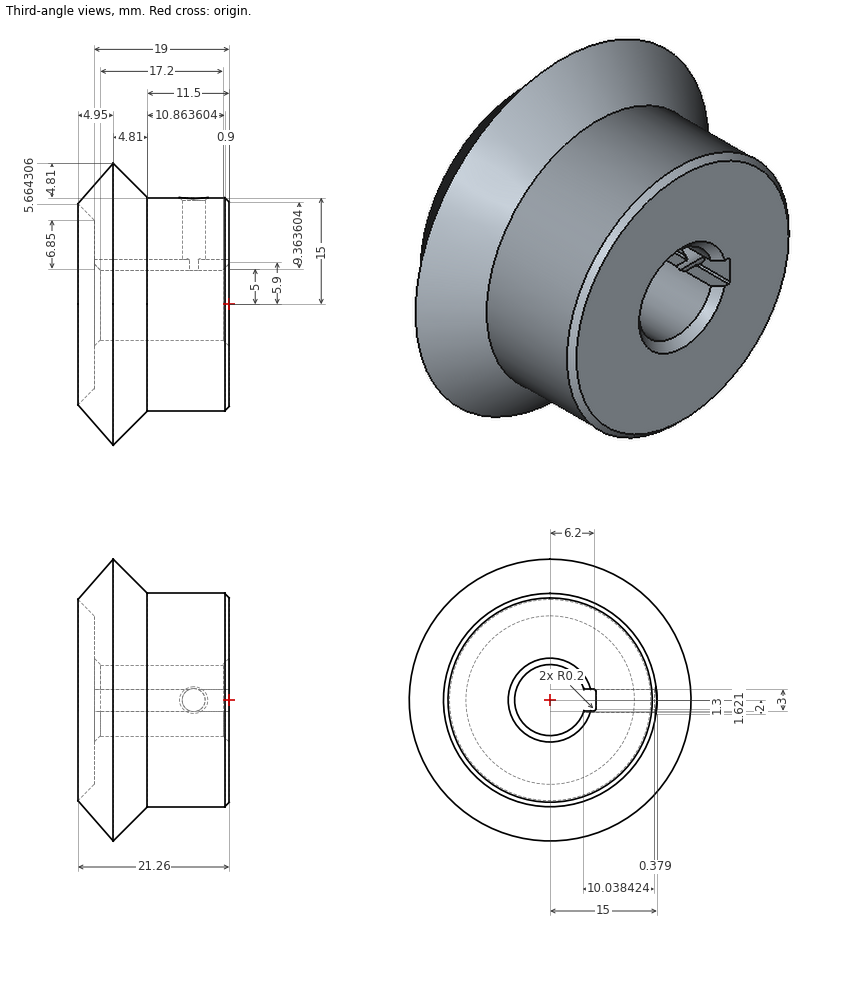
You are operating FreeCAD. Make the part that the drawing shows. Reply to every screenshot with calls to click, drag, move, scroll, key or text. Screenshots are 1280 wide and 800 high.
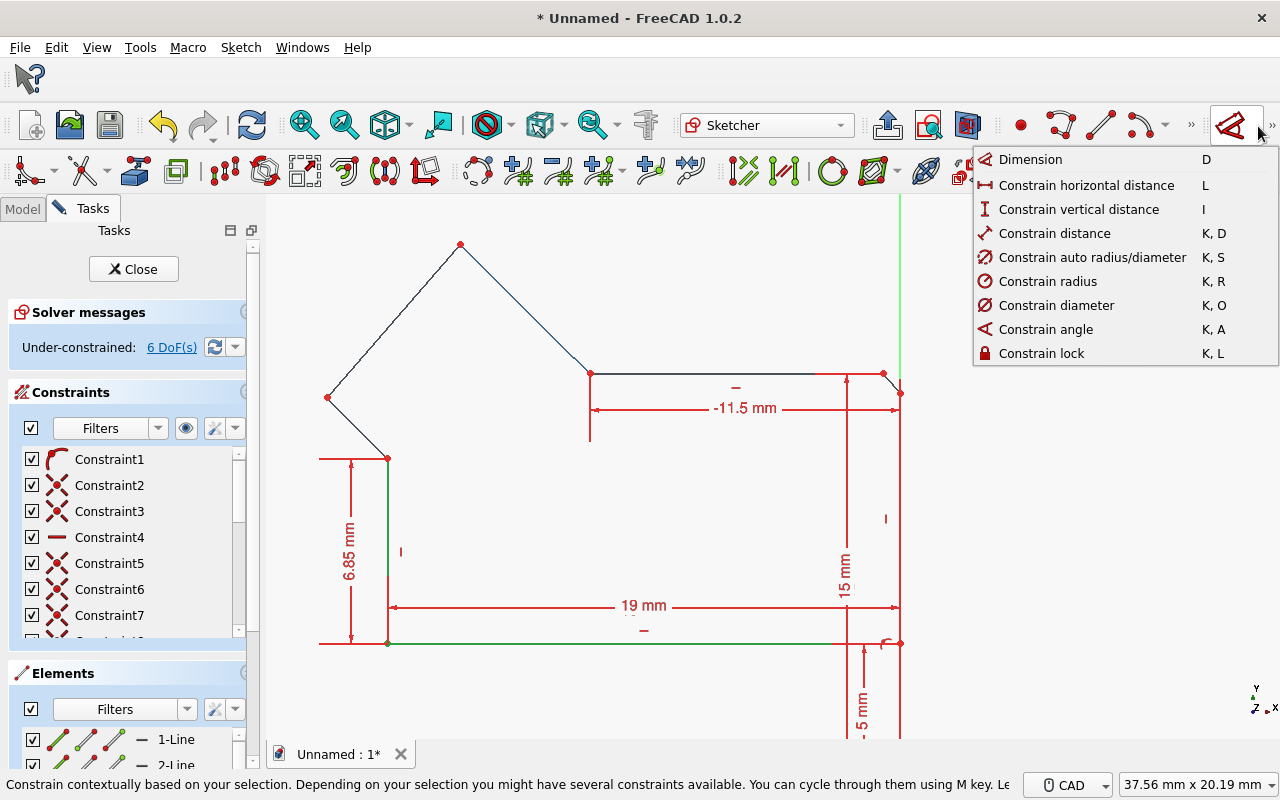
click(1126, 185)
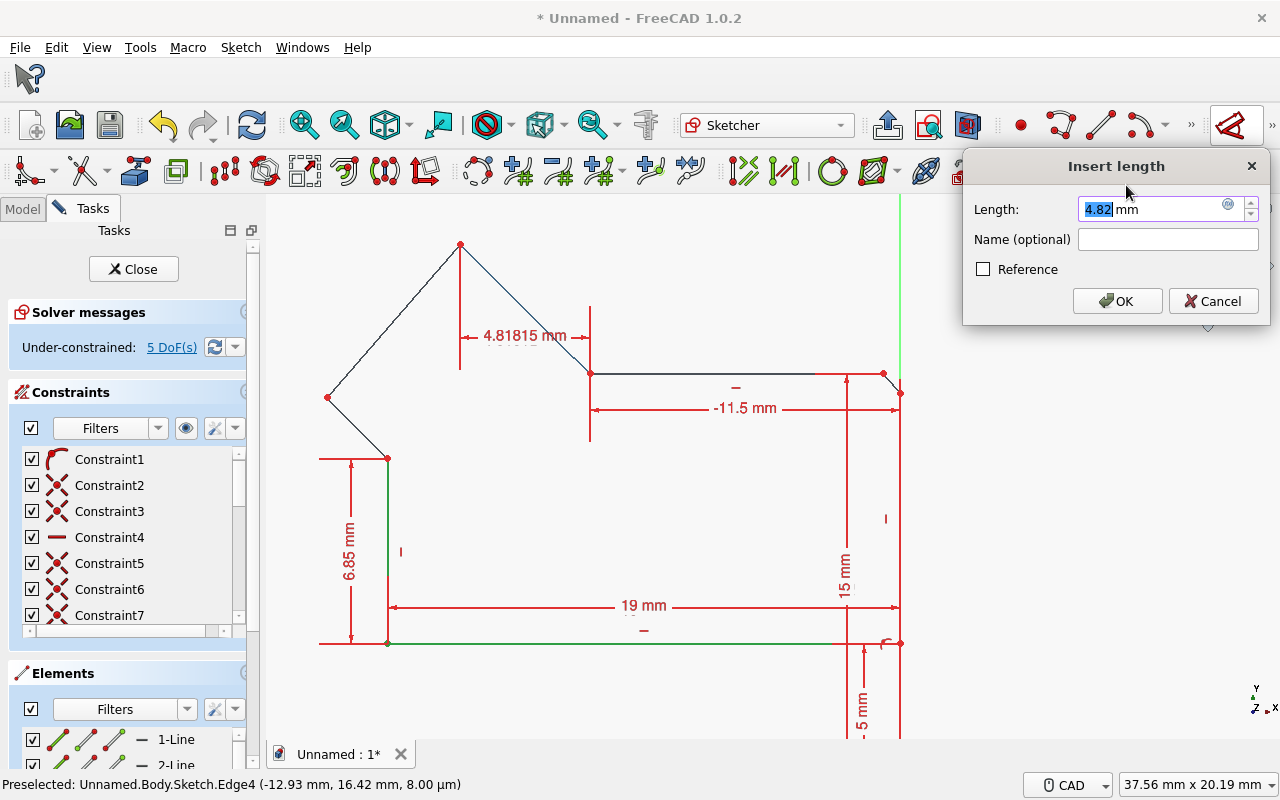
text(4.81)
key(Return)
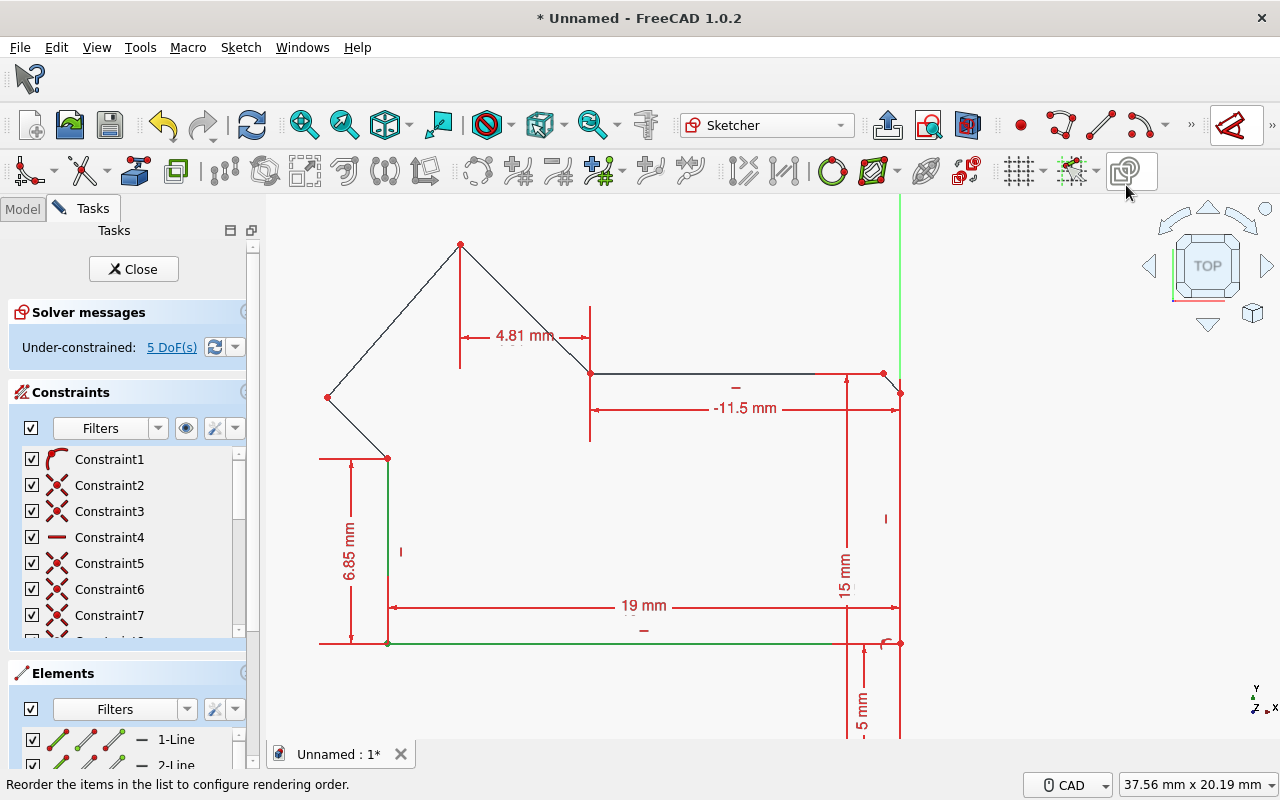
click(499, 284)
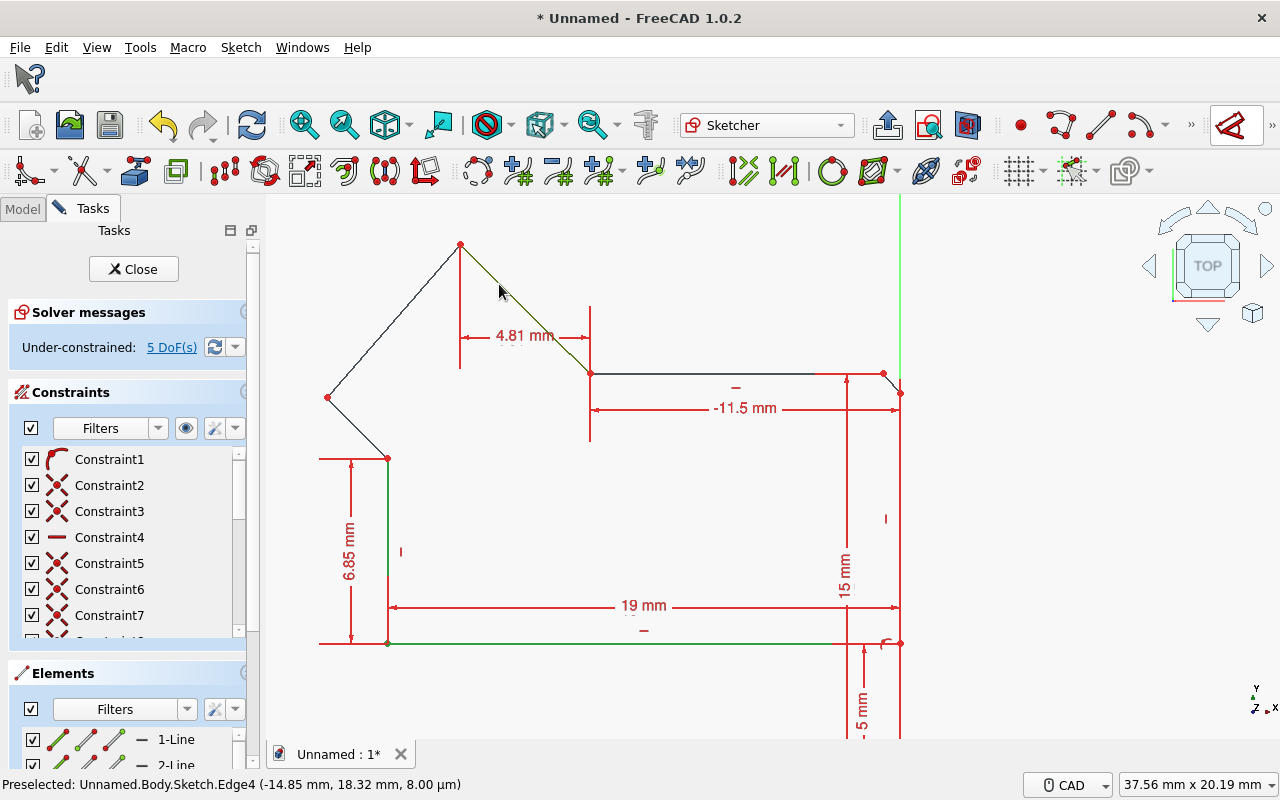
key(i)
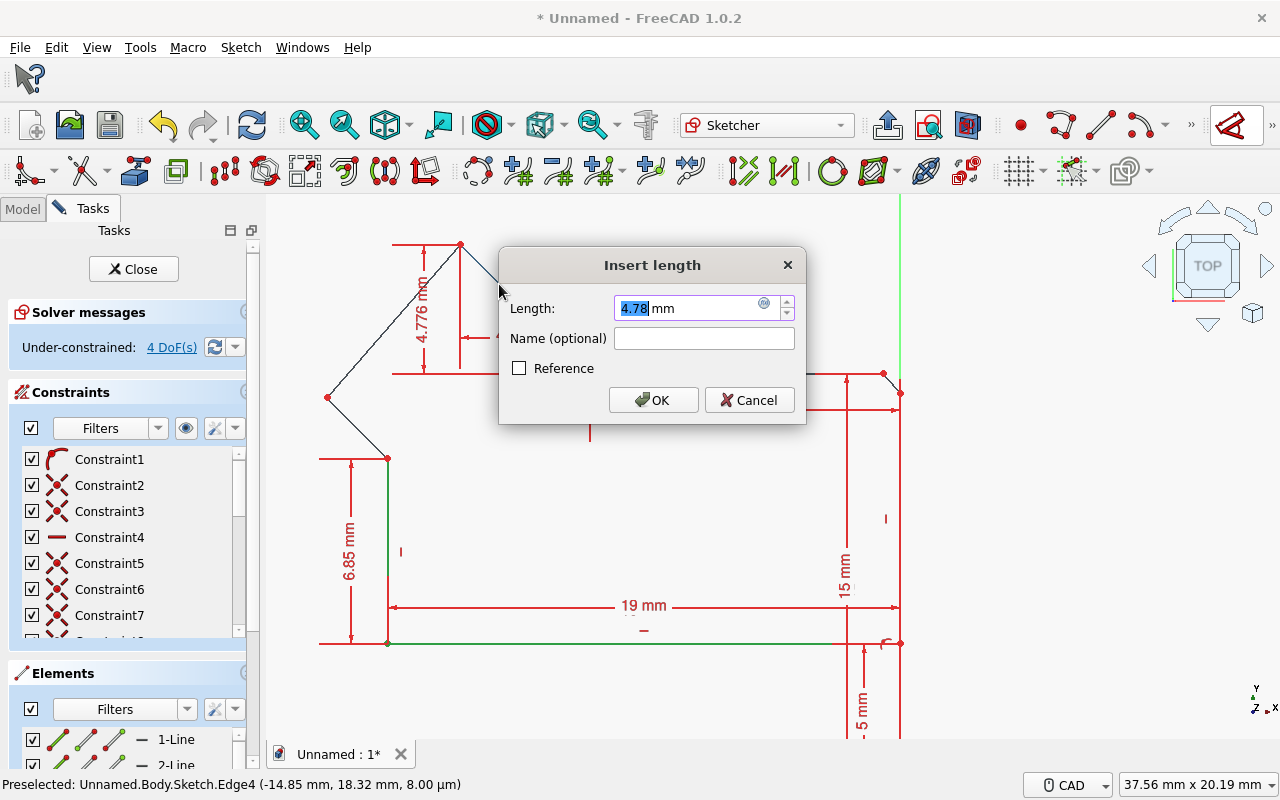
text(4.81)
key(Return)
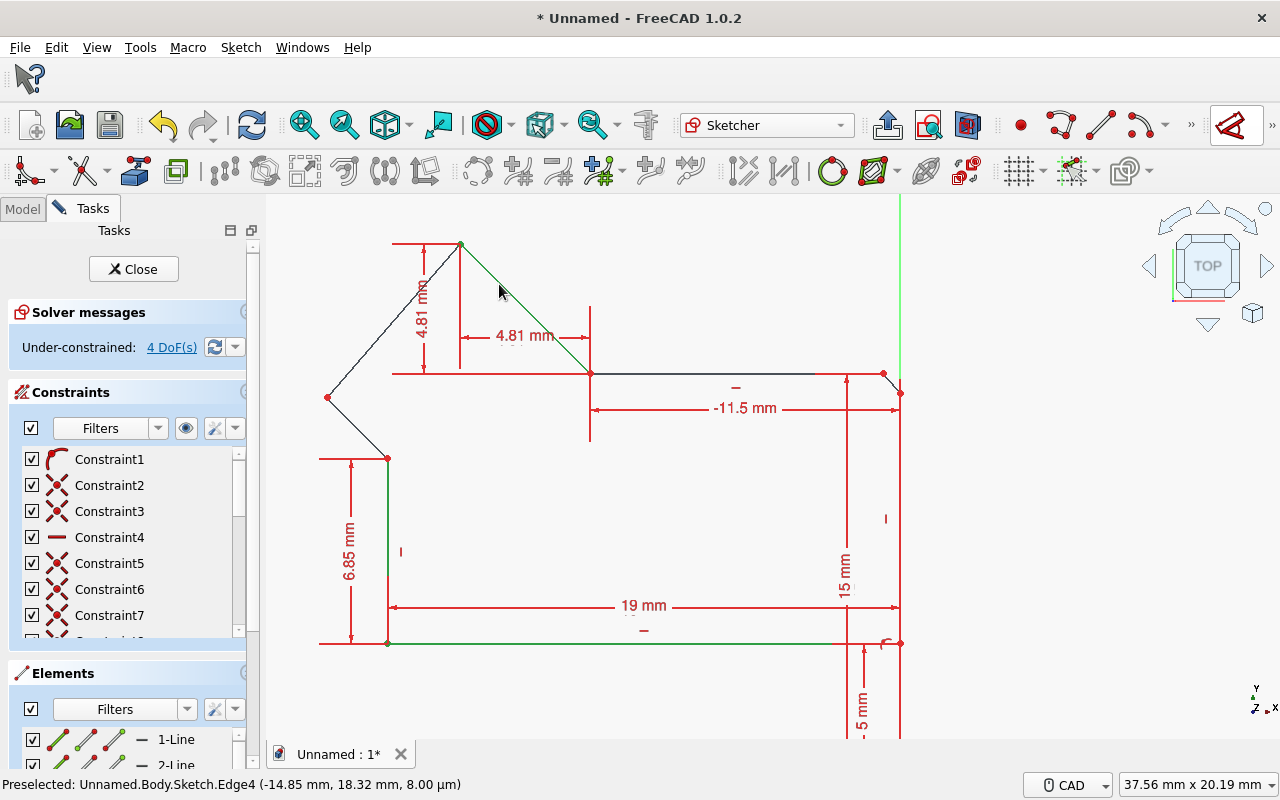
click(367, 352)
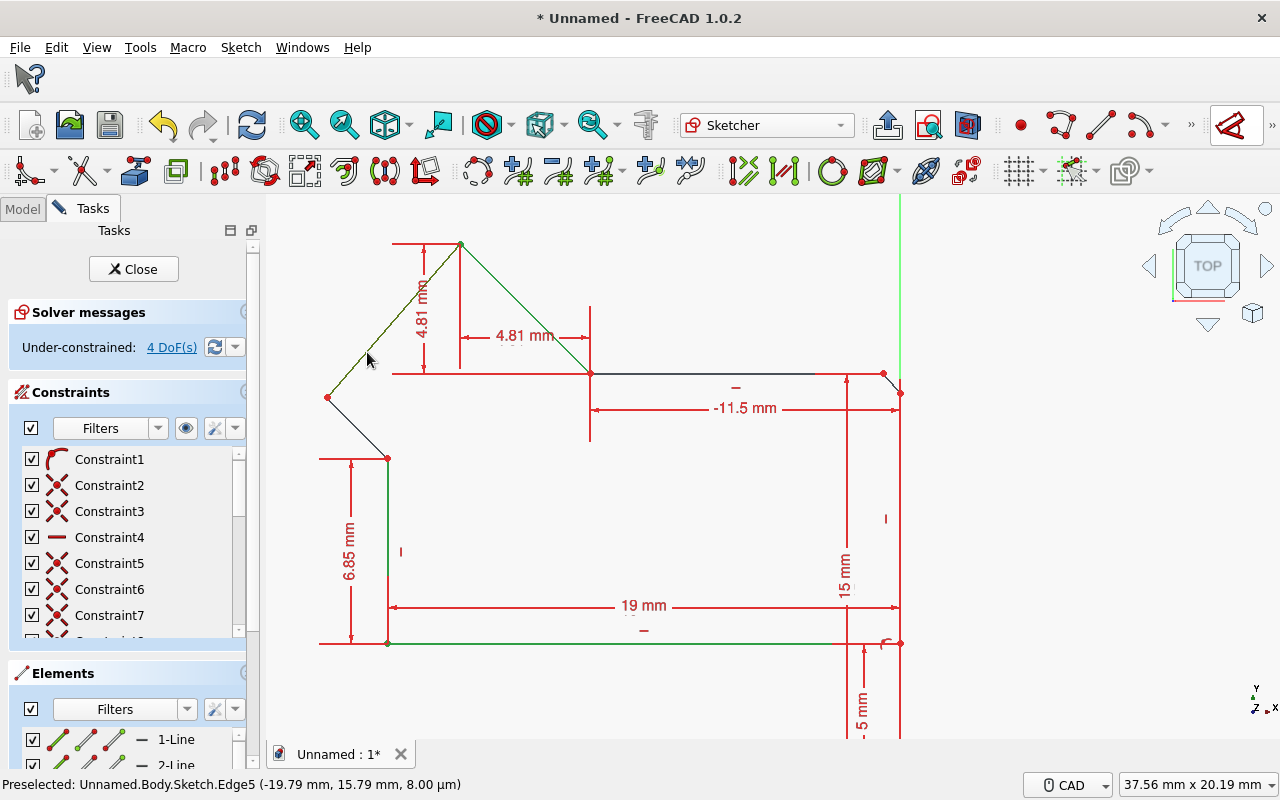
click(1258, 126)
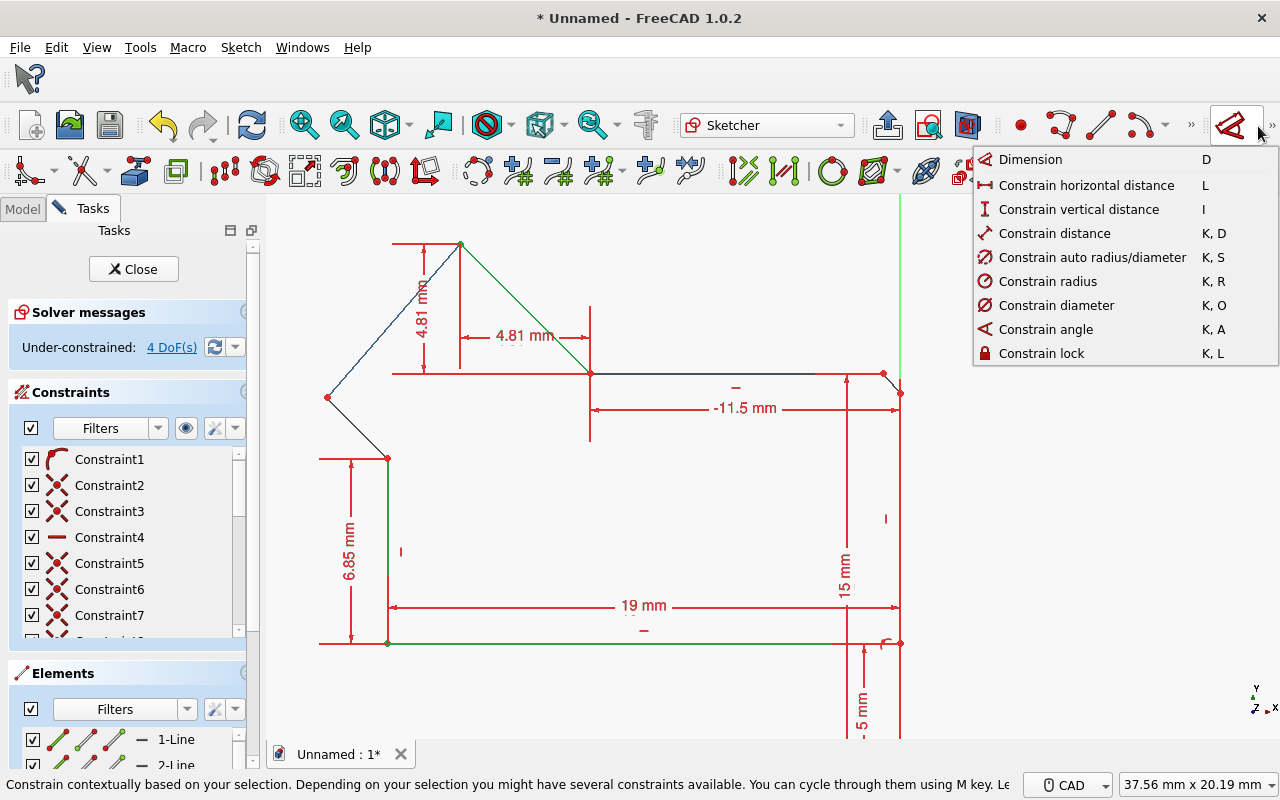
click(1126, 185)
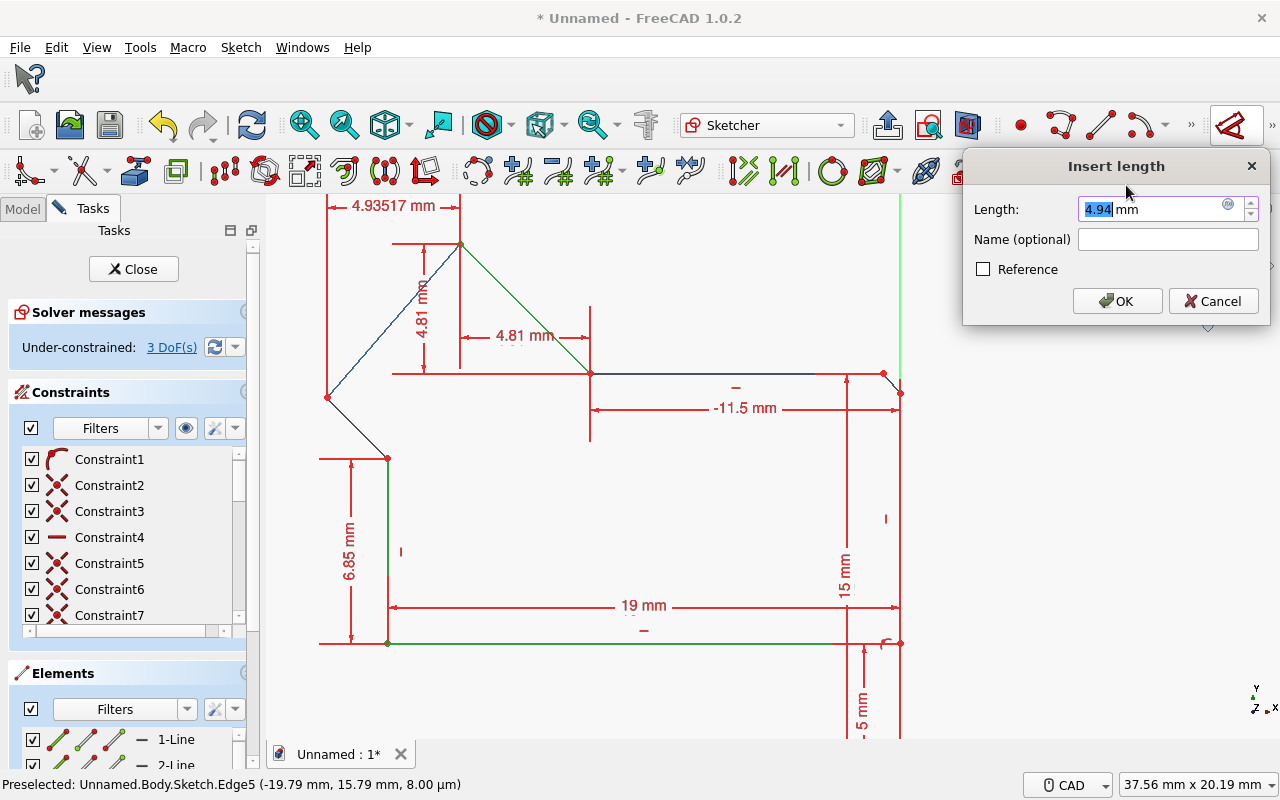
text(4.95)
key(Return)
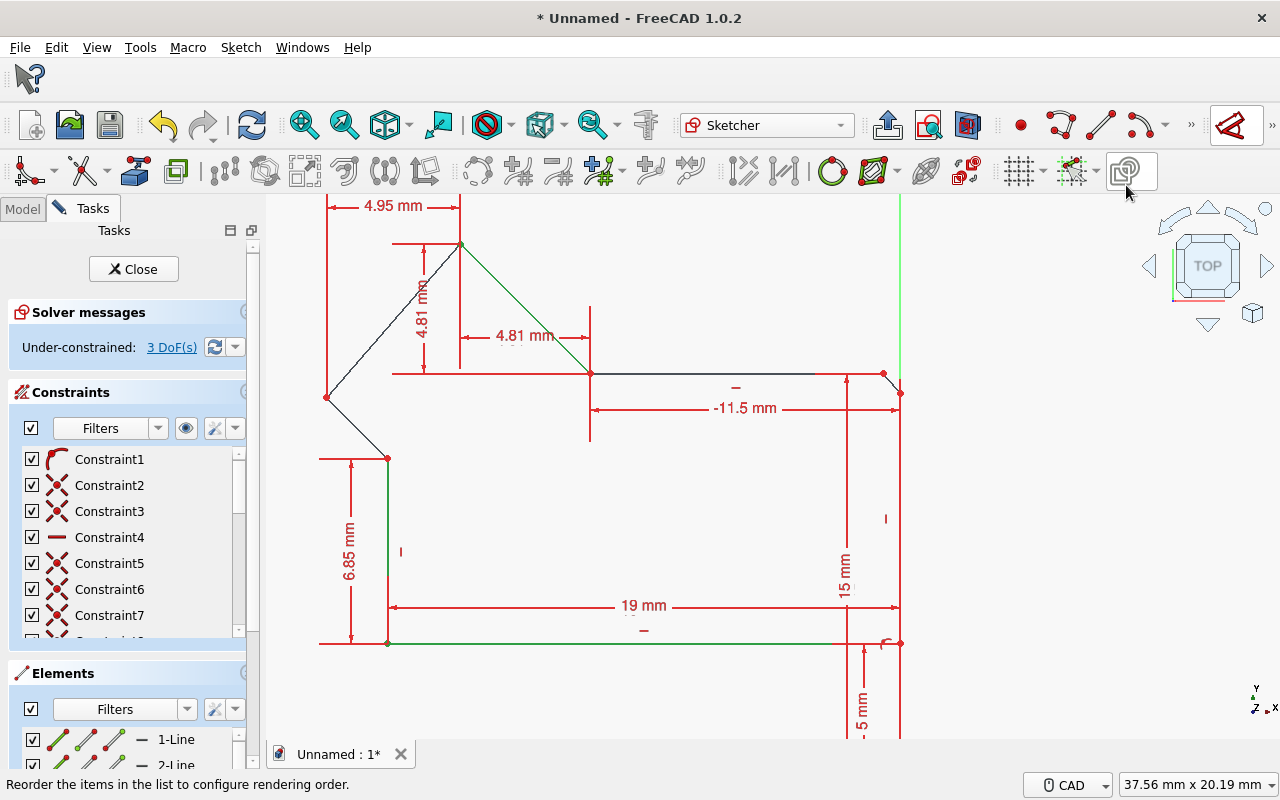
click(900, 569)